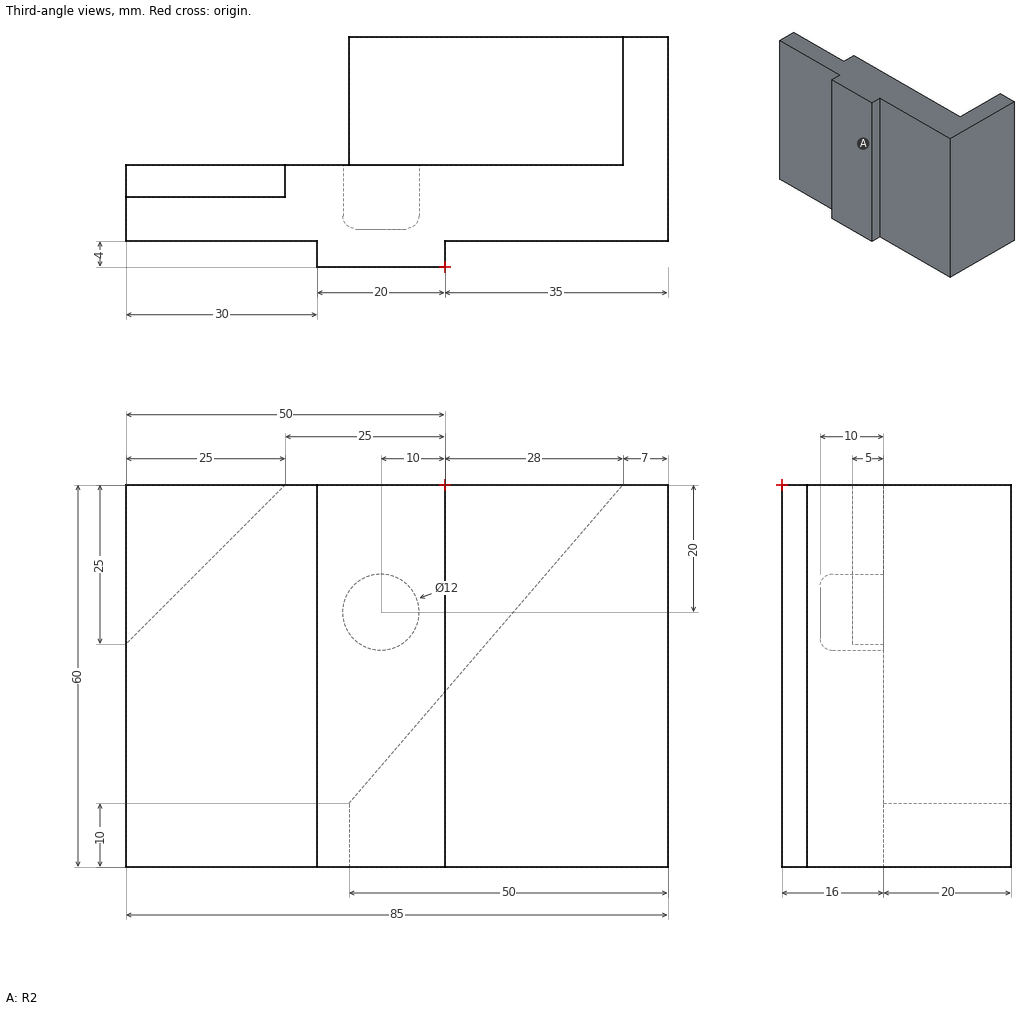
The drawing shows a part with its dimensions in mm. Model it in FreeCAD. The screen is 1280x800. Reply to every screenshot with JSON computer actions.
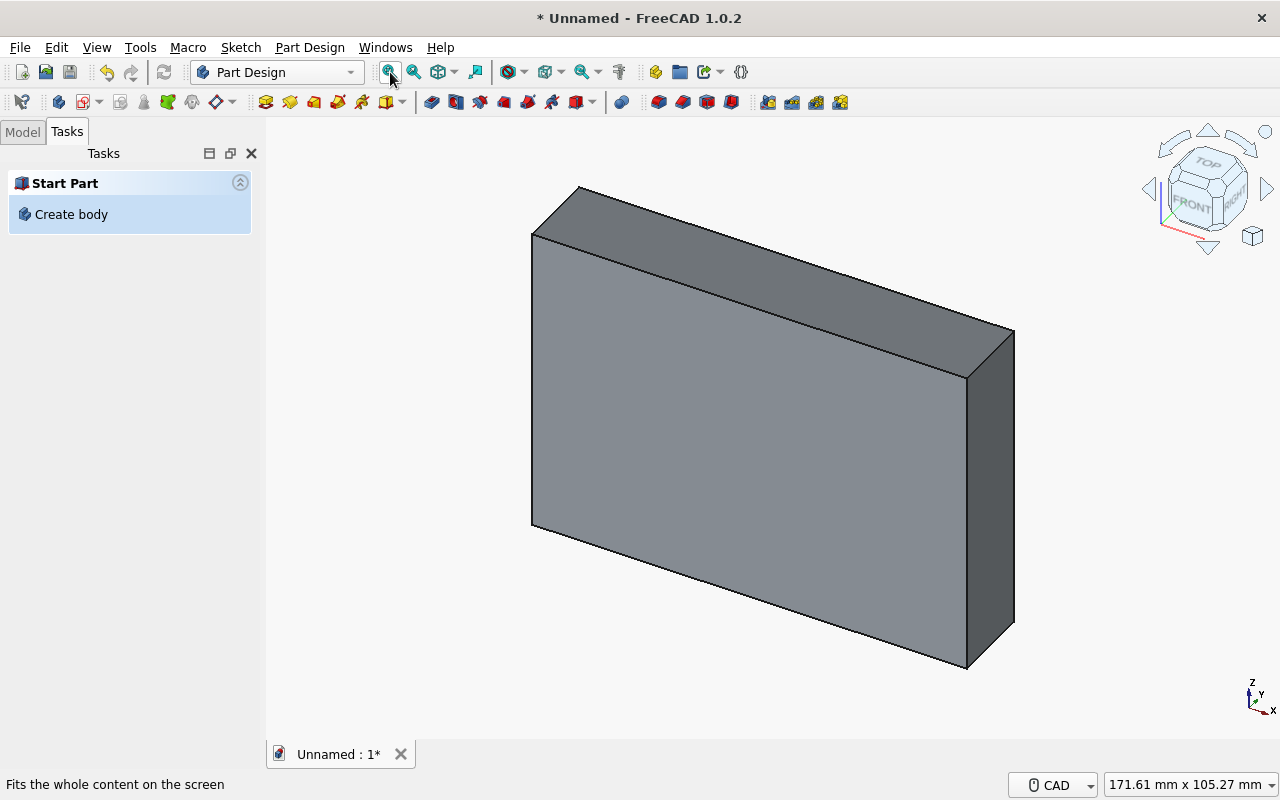
{"action": "left_click", "coordinate": [897, 323]}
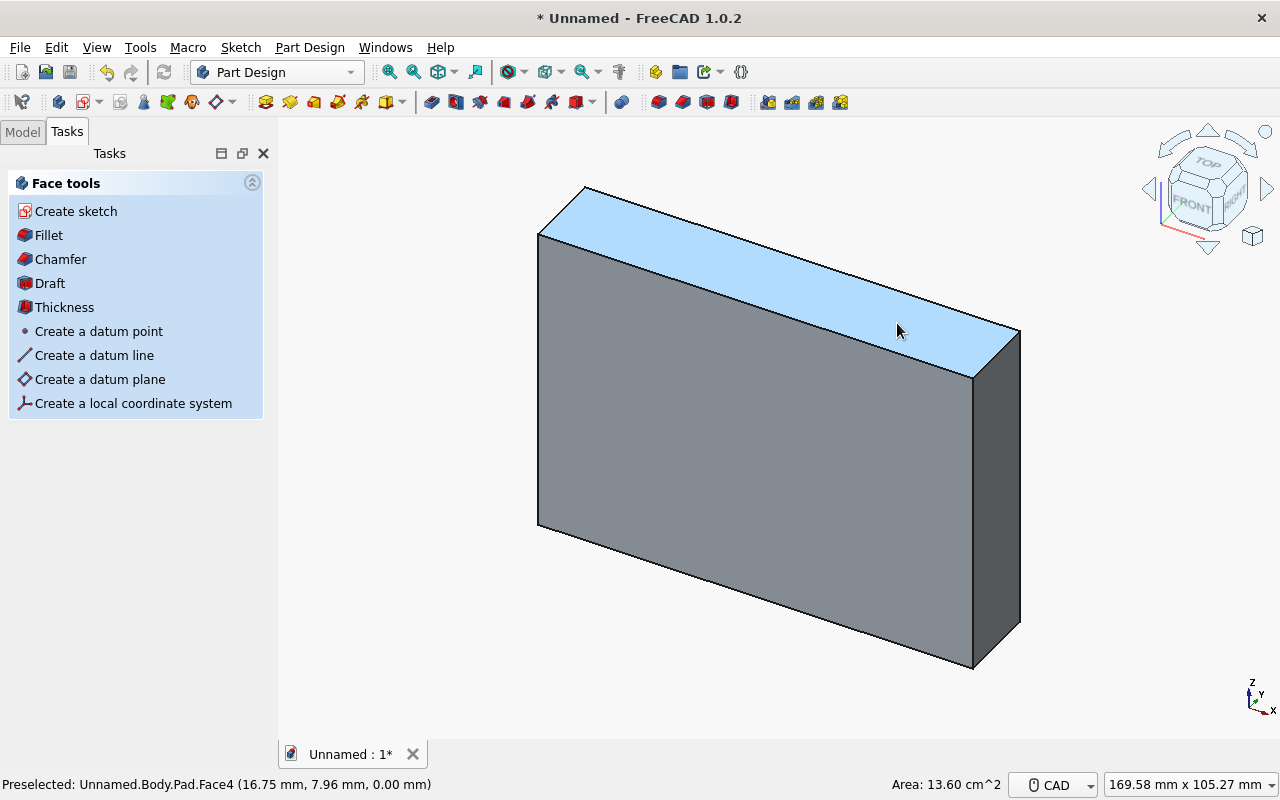
{"action": "left_click", "coordinate": [84, 102]}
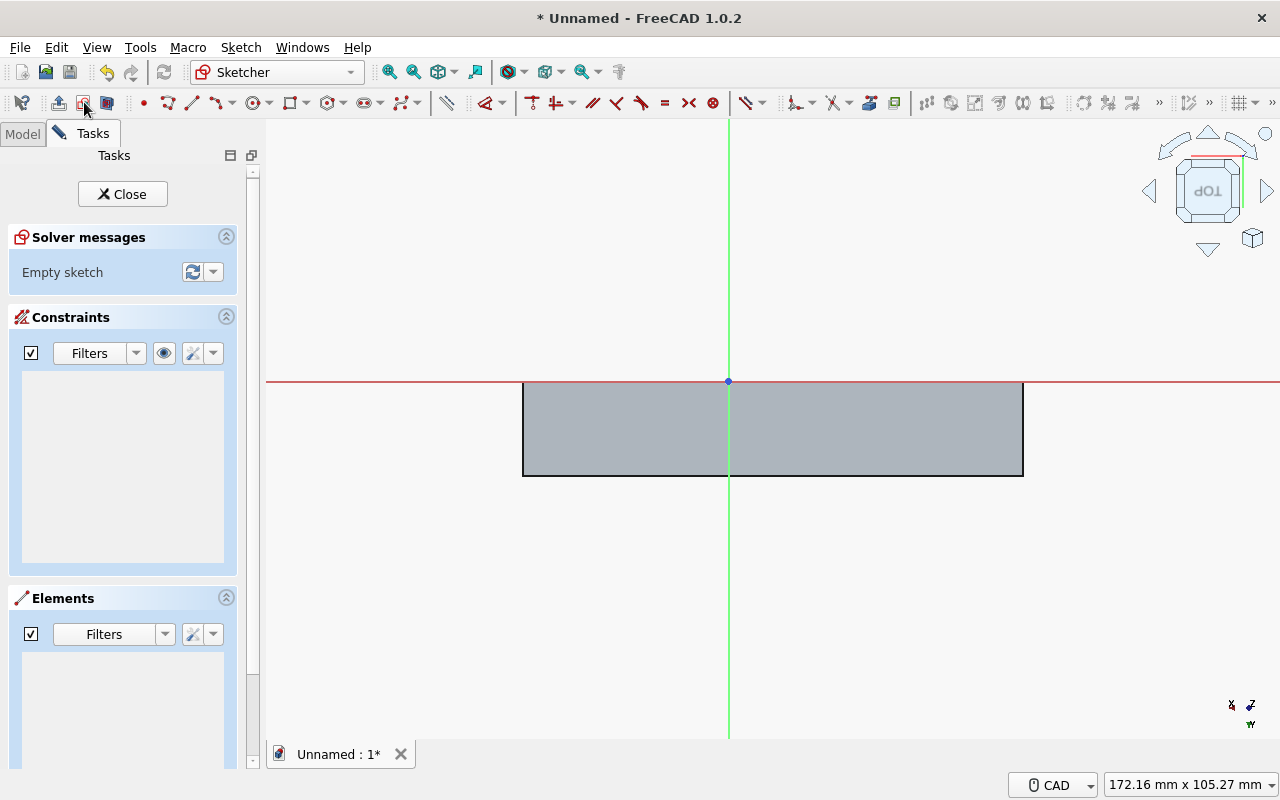
{"action": "scroll", "coordinate": [1085, 351], "scroll_direction": "up", "scroll_amount": 3}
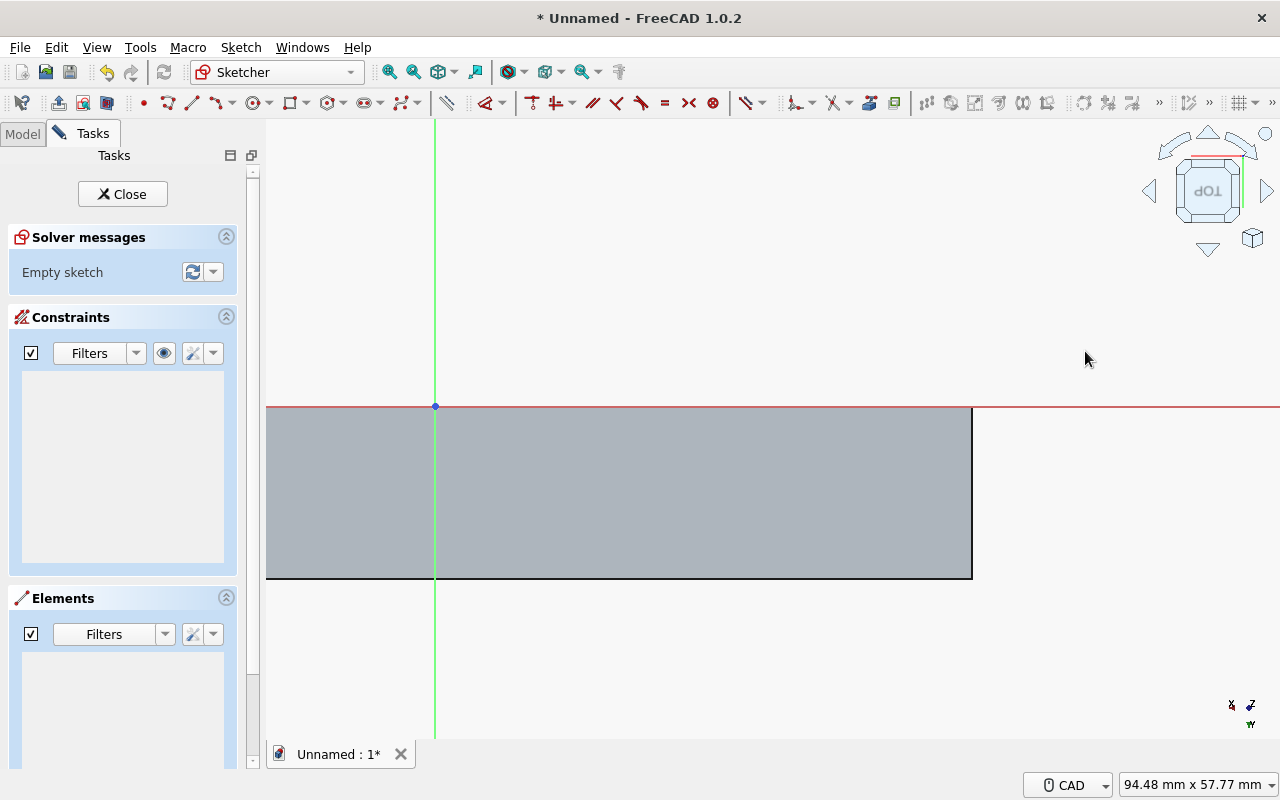
{"action": "left_click", "coordinate": [290, 104]}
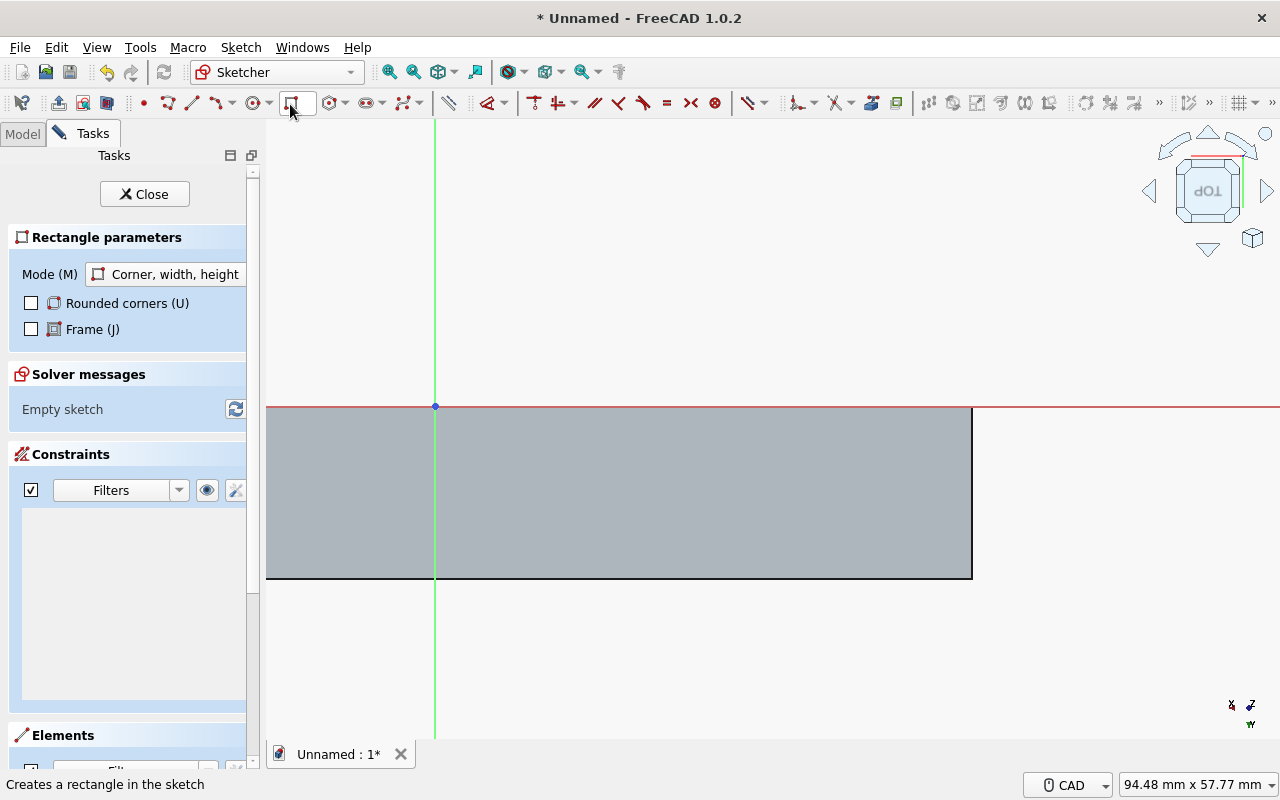
{"action": "left_click", "coordinate": [650, 407]}
{"action": "left_click", "coordinate": [972, 450]}
{"action": "key", "text": "Escape"}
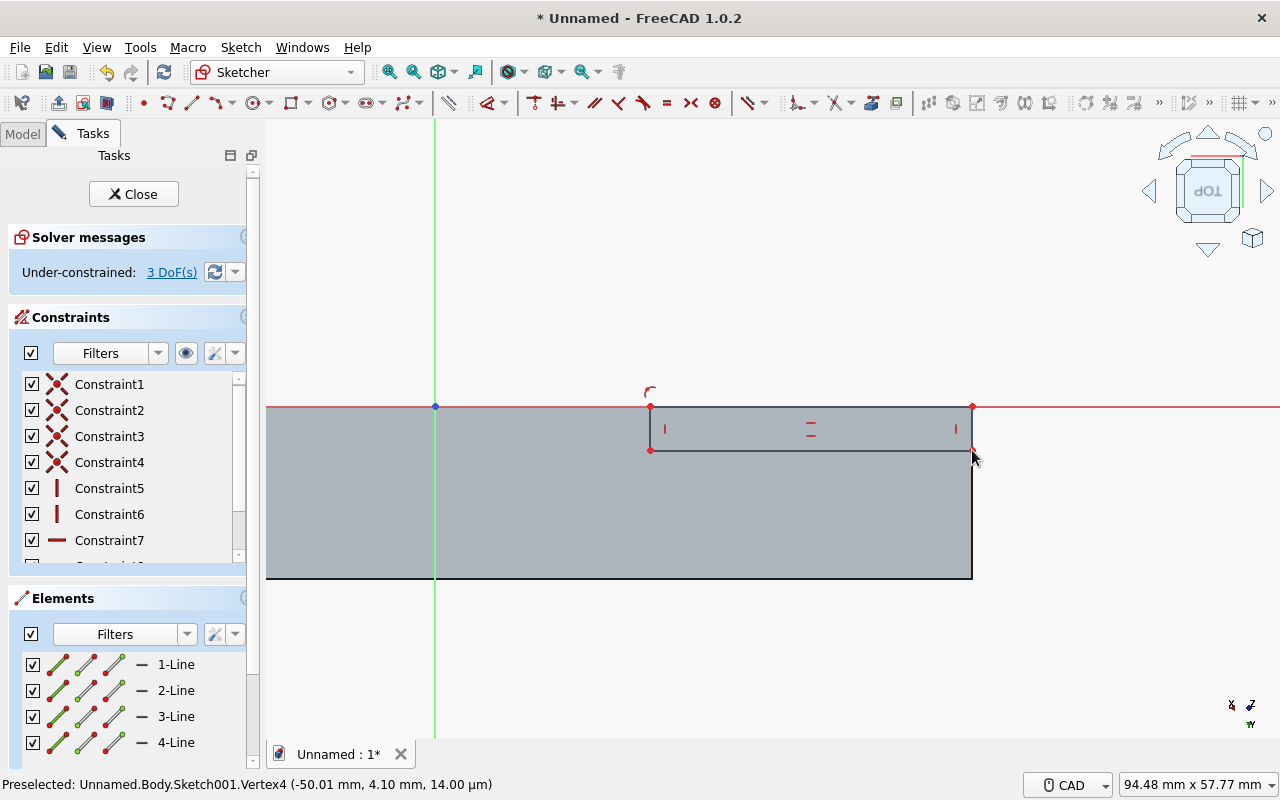
{"action": "left_click", "coordinate": [488, 104]}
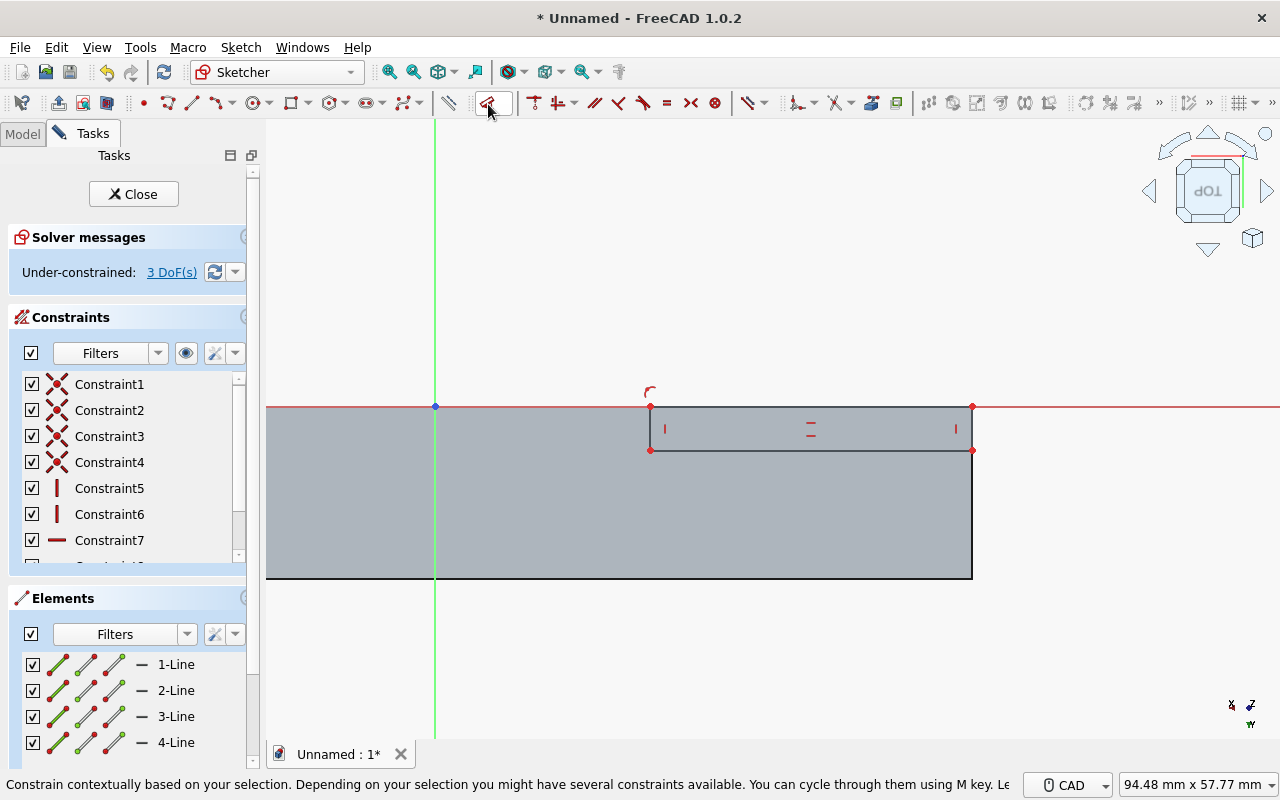
{"action": "left_click", "coordinate": [650, 420]}
{"action": "left_click", "coordinate": [616, 429]}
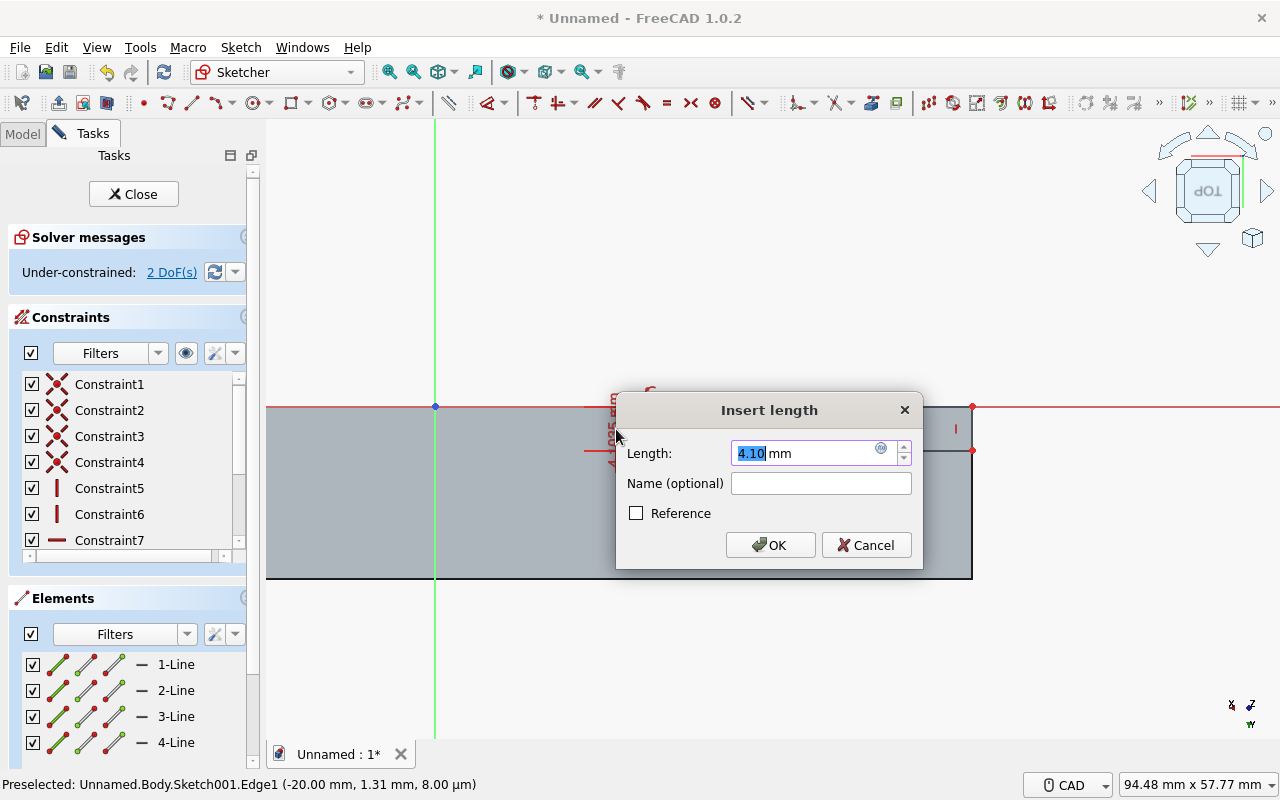
{"action": "type", "text": "4"}
{"action": "key", "text": "Return"}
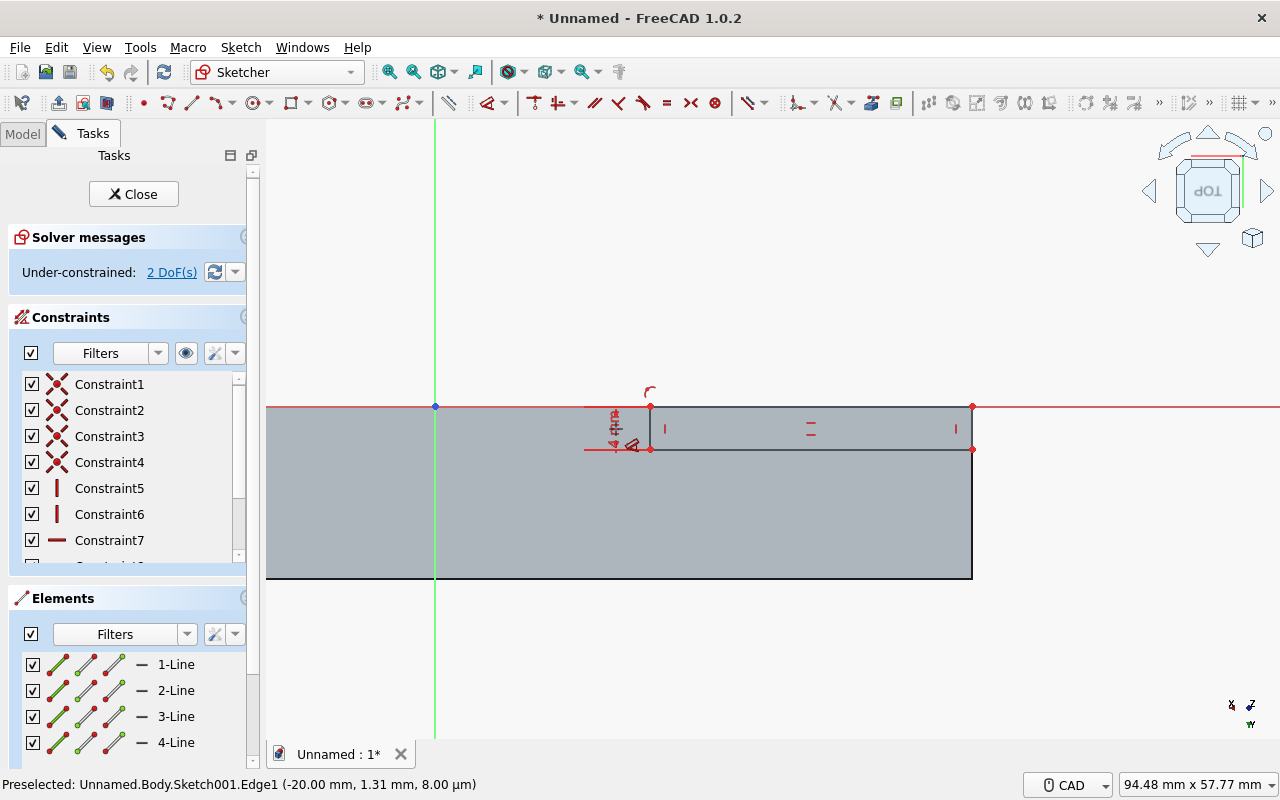
{"action": "left_click", "coordinate": [747, 450]}
{"action": "left_click", "coordinate": [811, 484]}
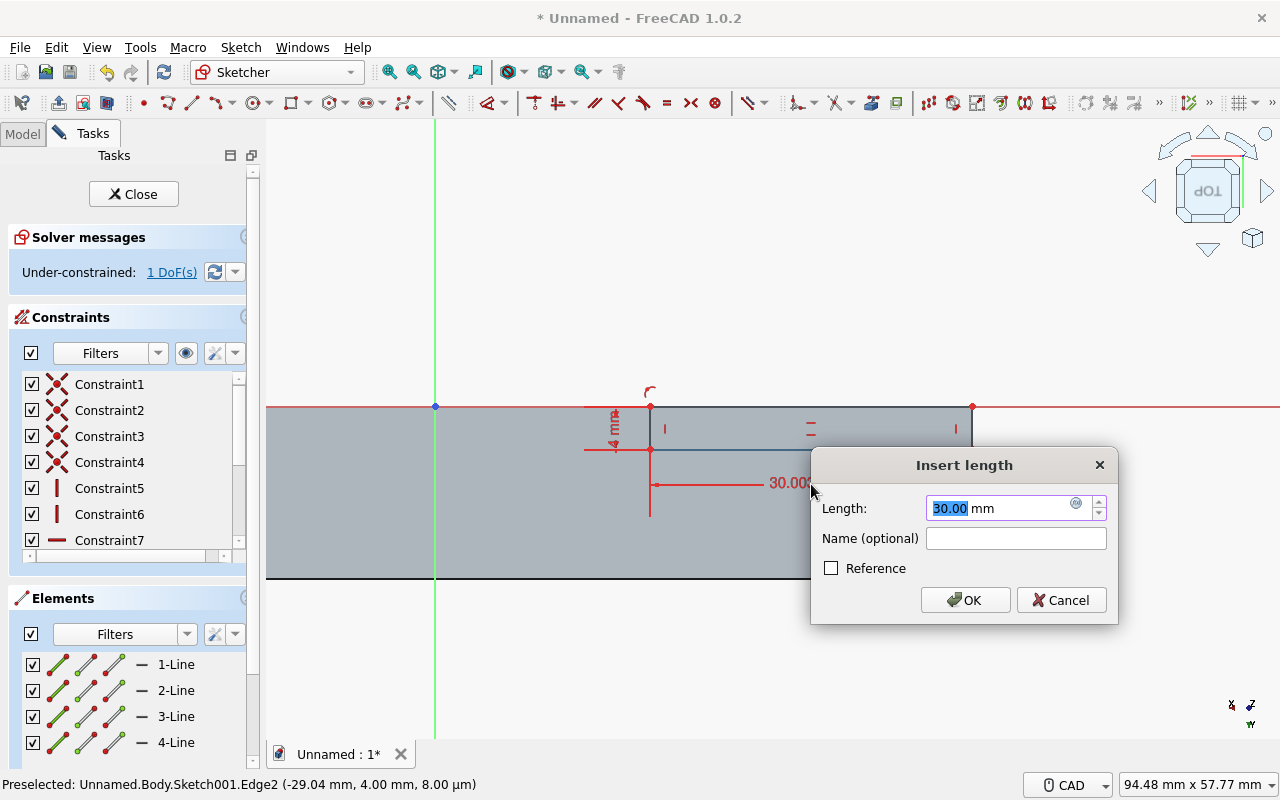
{"action": "type", "text": "30"}
{"action": "key", "text": "Return"}